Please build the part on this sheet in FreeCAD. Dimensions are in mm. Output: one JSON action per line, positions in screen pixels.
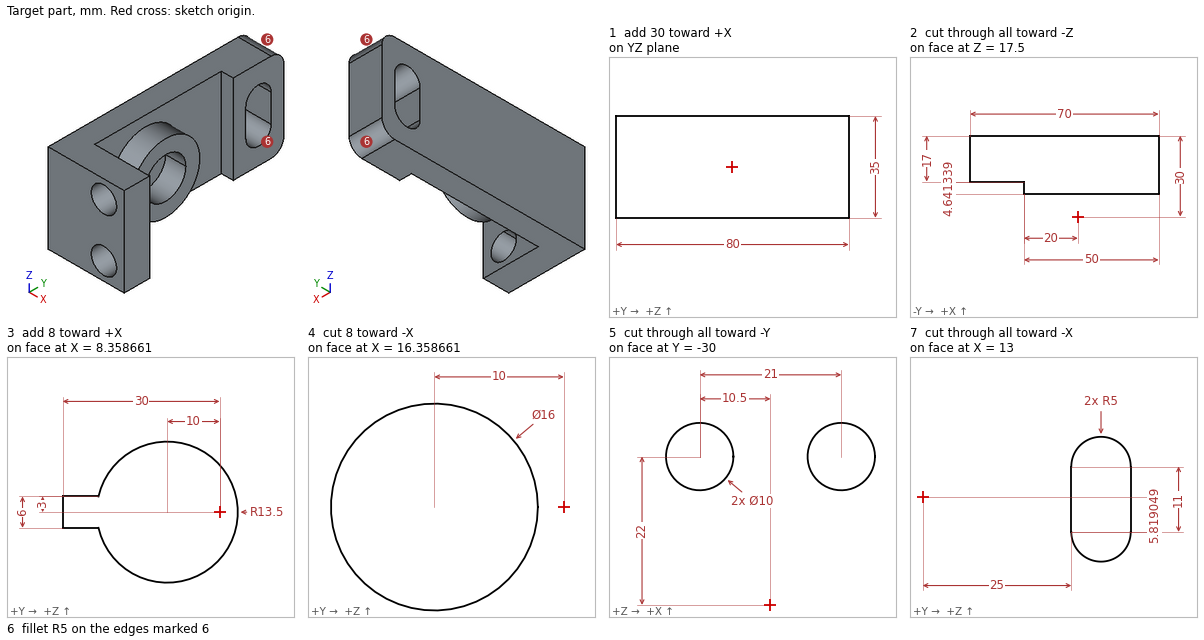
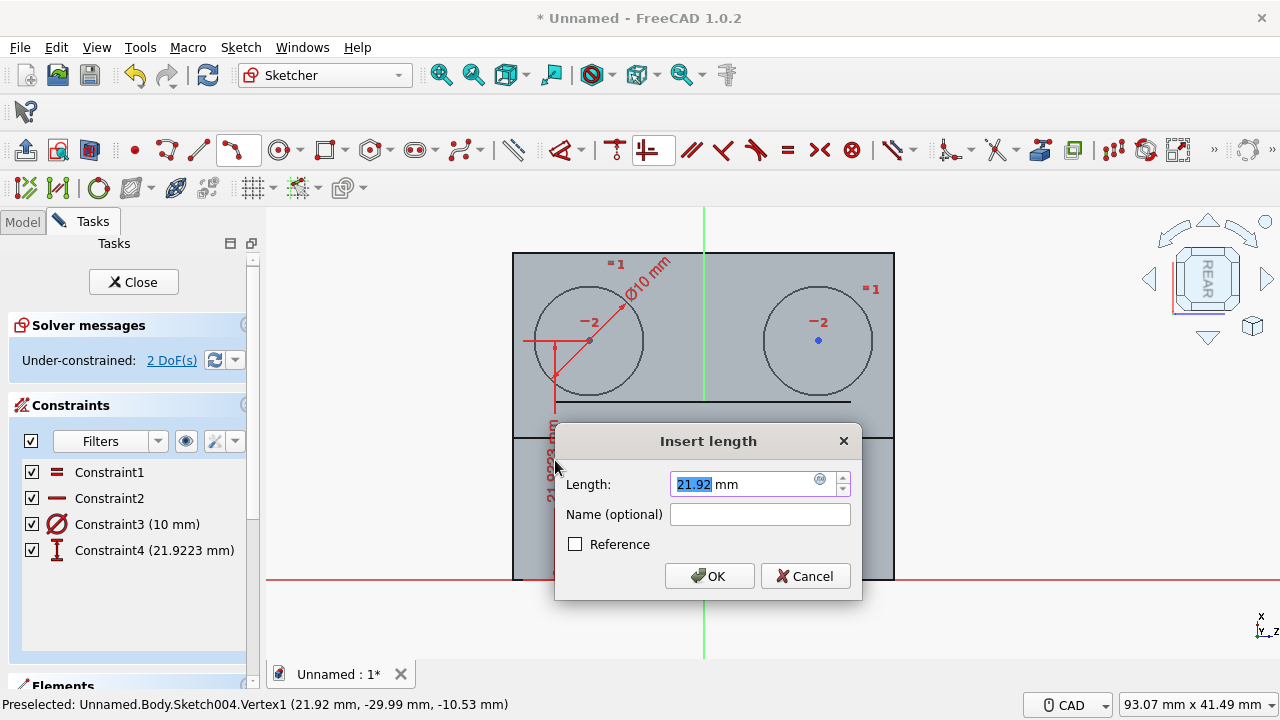
{"action": "type", "text": "22"}
{"action": "key", "text": "Return"}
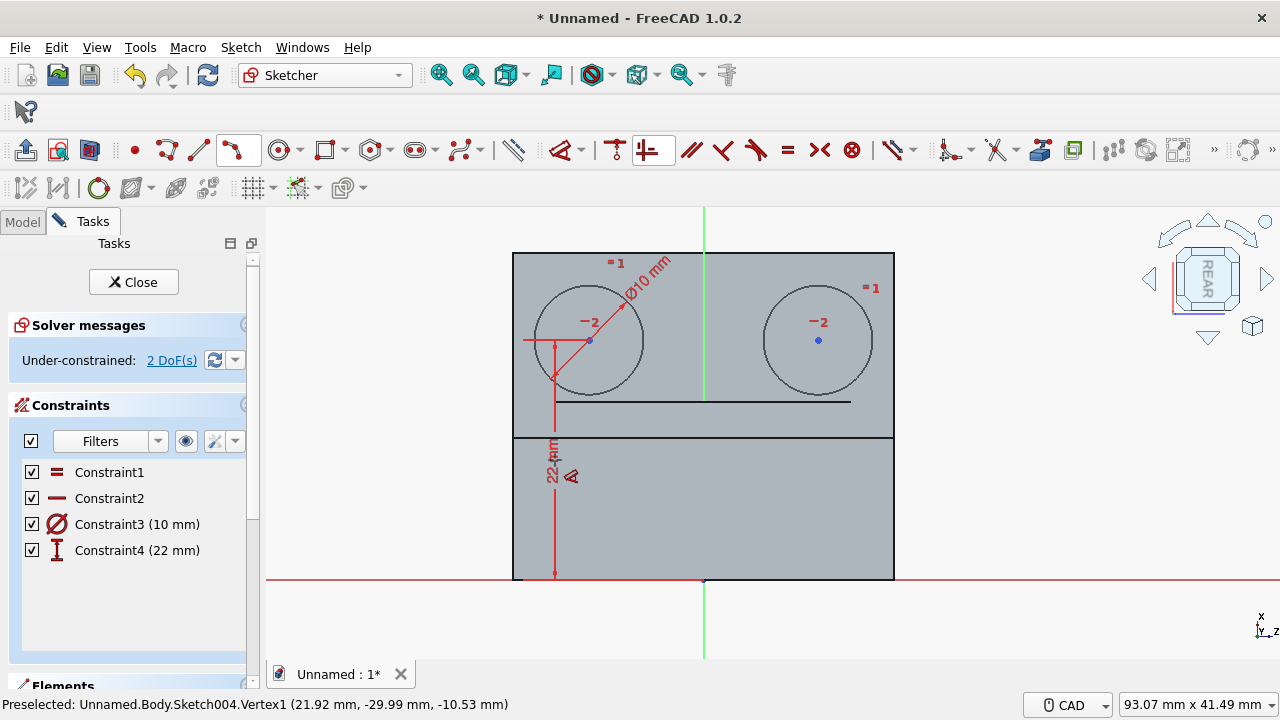
{"action": "left_click", "coordinate": [589, 340]}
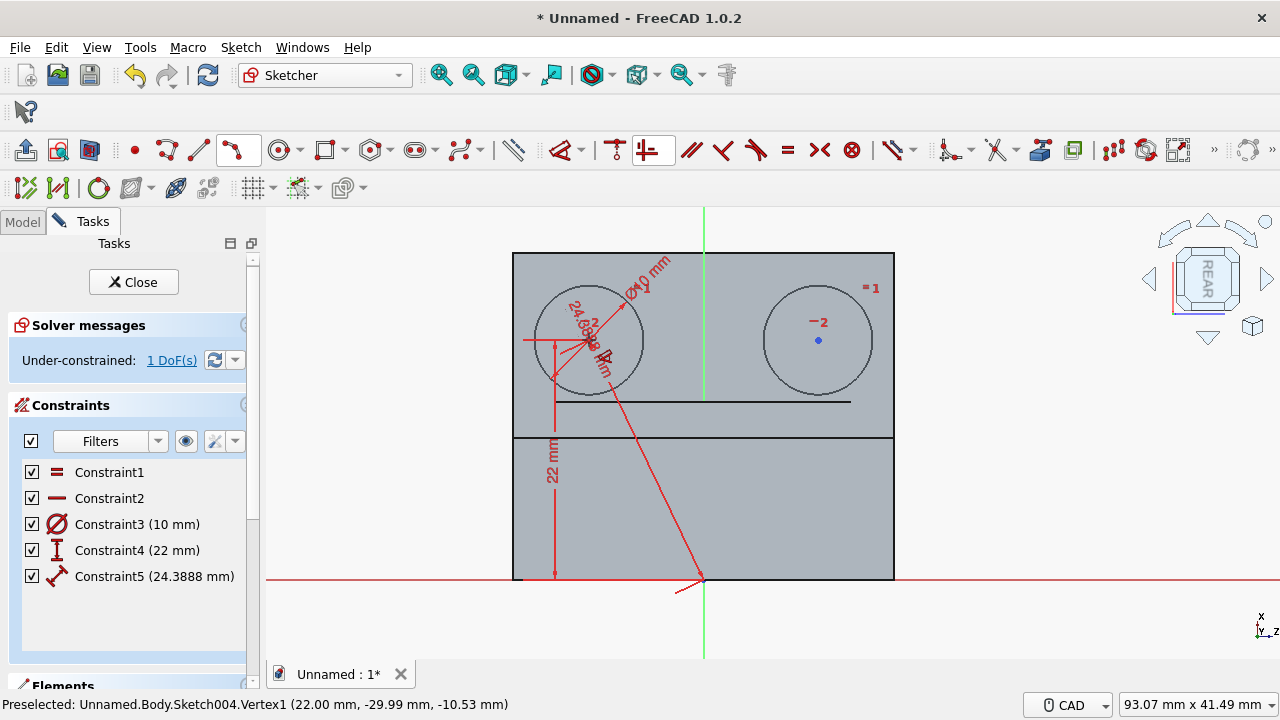
{"action": "left_click", "coordinate": [818, 340]}
{"action": "left_click", "coordinate": [651, 306]}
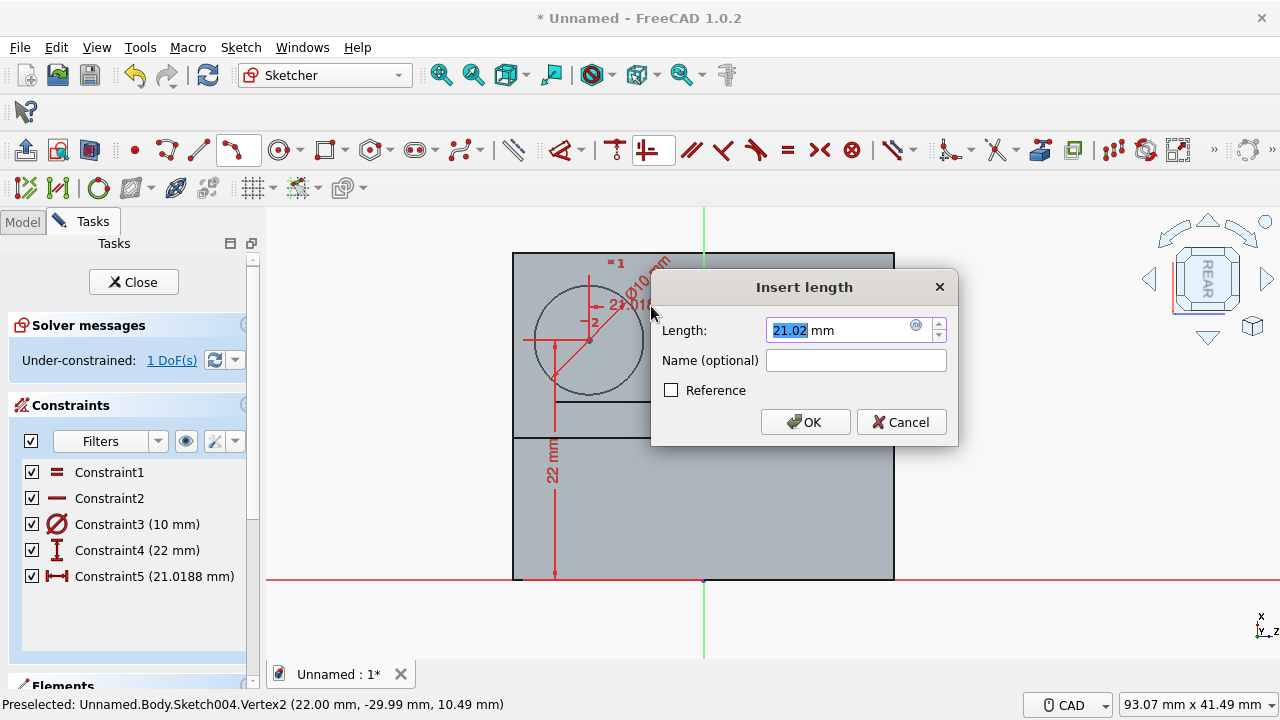
{"action": "type", "text": "21"}
{"action": "key", "text": "Return"}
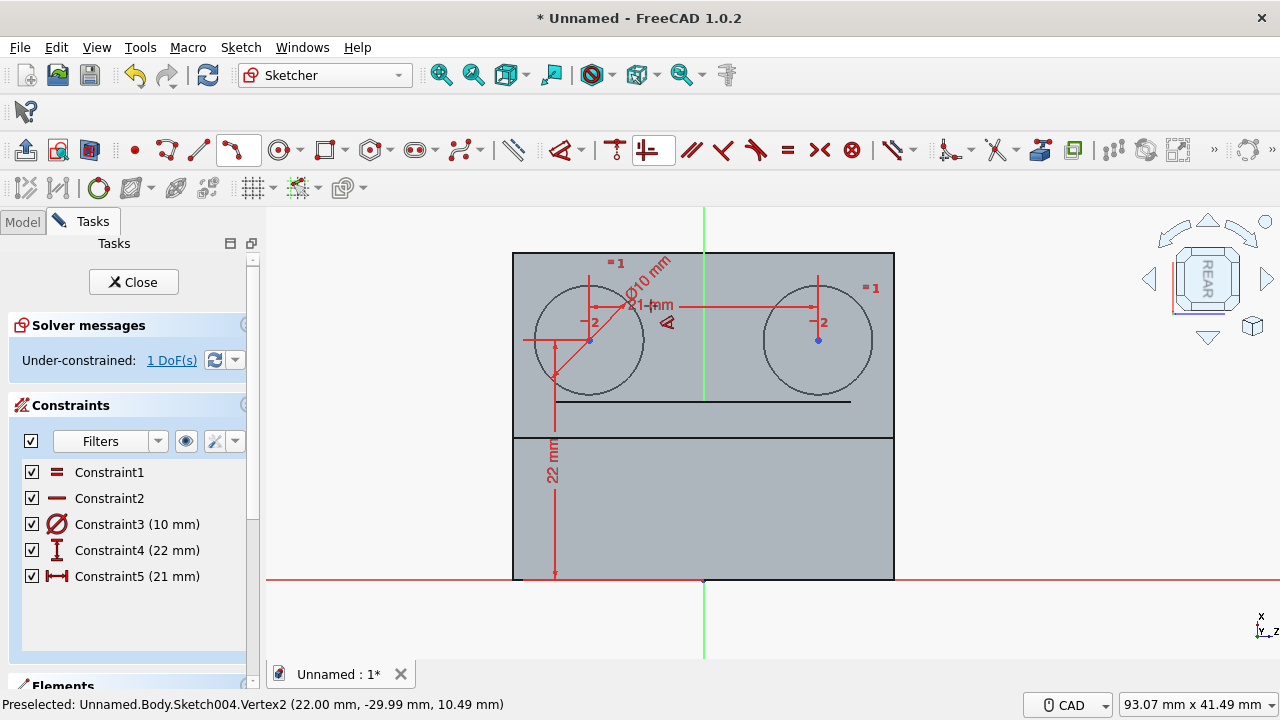
{"action": "left_click", "coordinate": [589, 340]}
{"action": "left_click", "coordinate": [646, 614]}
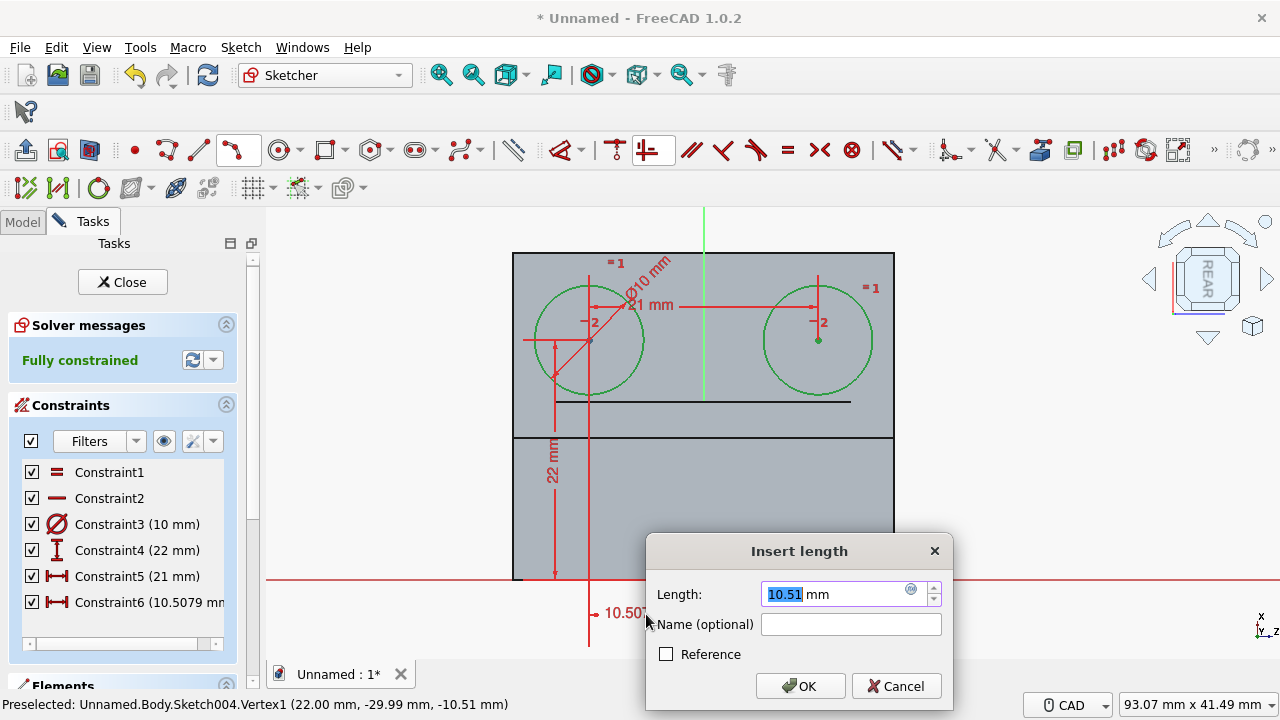
{"action": "type", "text": "10.5"}
{"action": "key", "text": "Return"}
{"action": "key", "text": "Escape"}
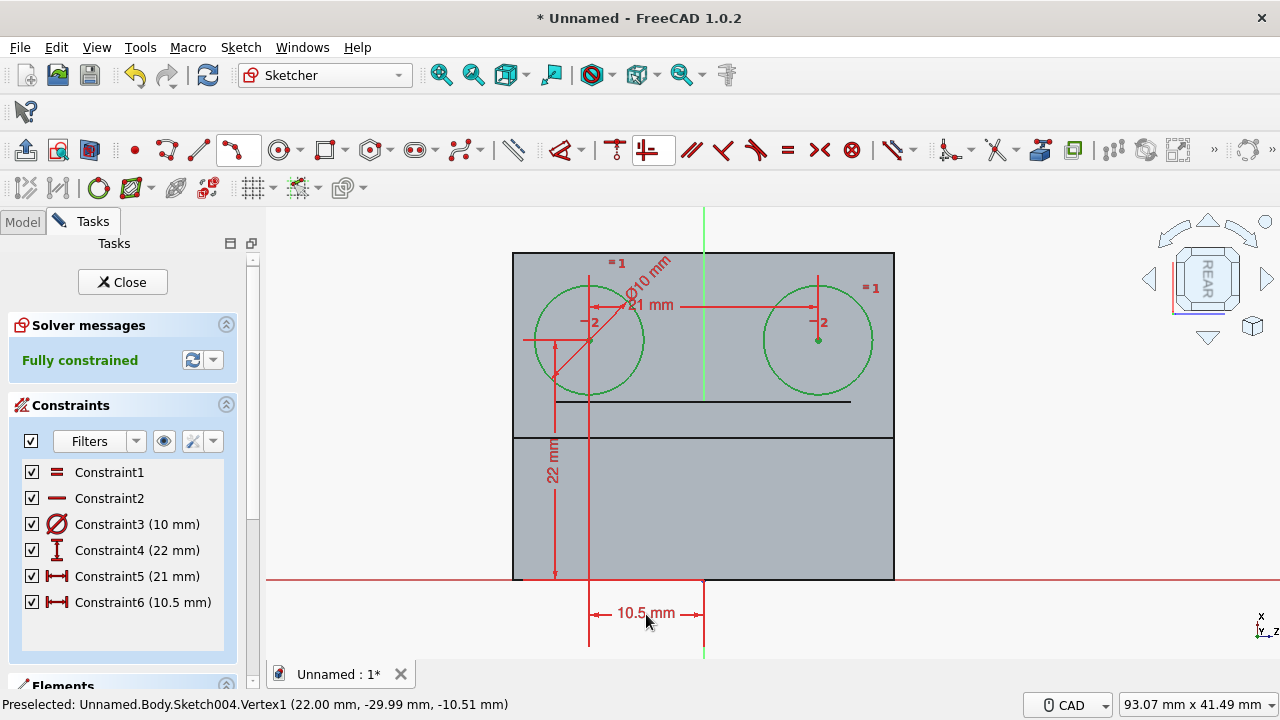
{"action": "left_click", "coordinate": [123, 282]}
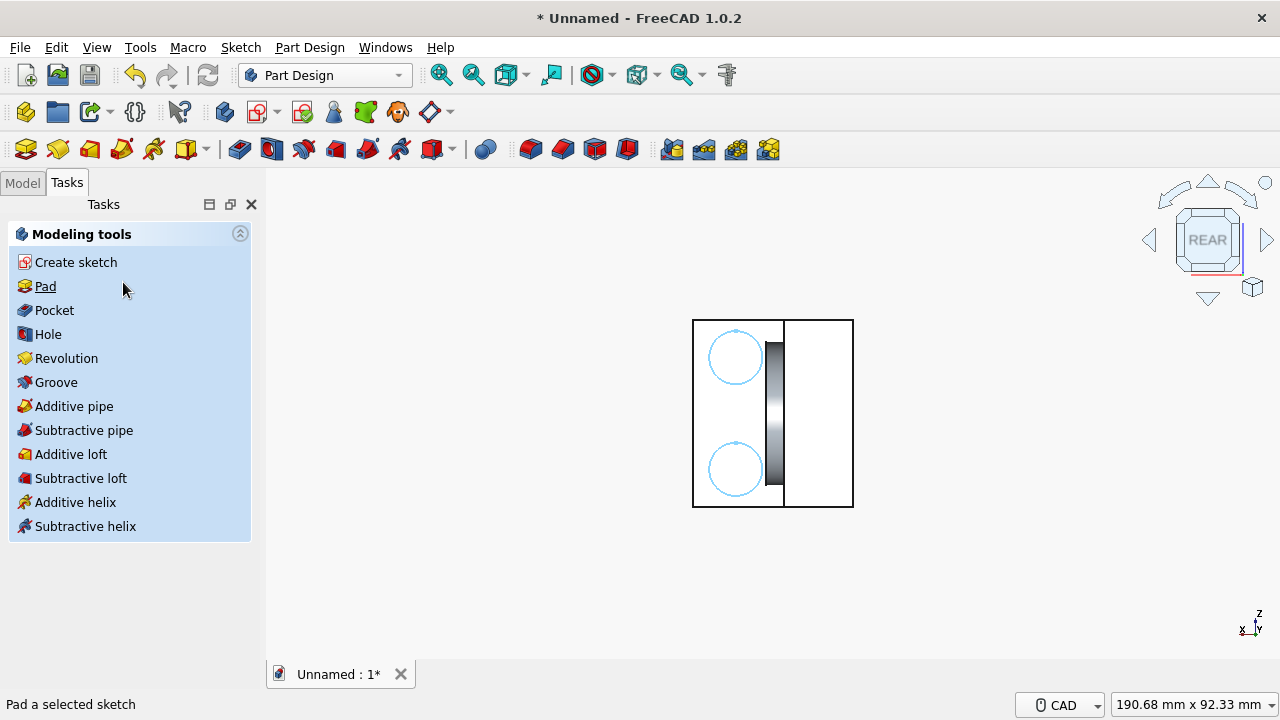
{"action": "left_click", "coordinate": [240, 150]}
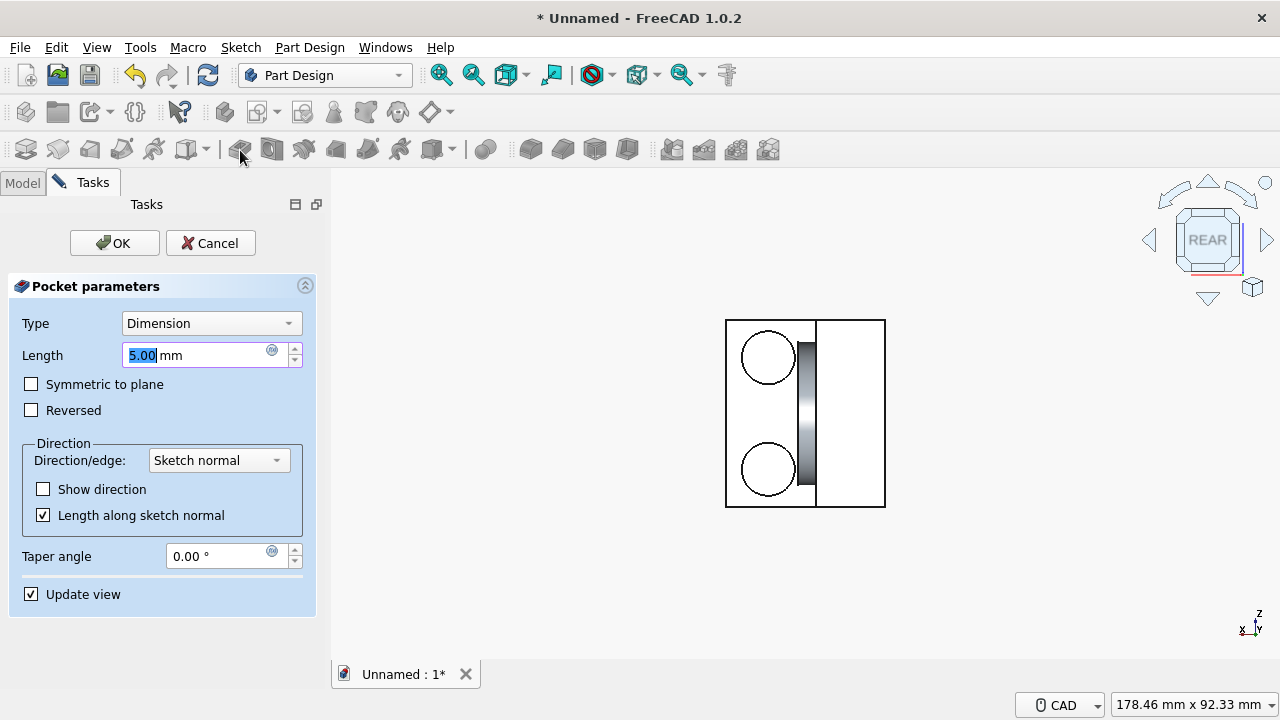
{"action": "left_click", "coordinate": [212, 324]}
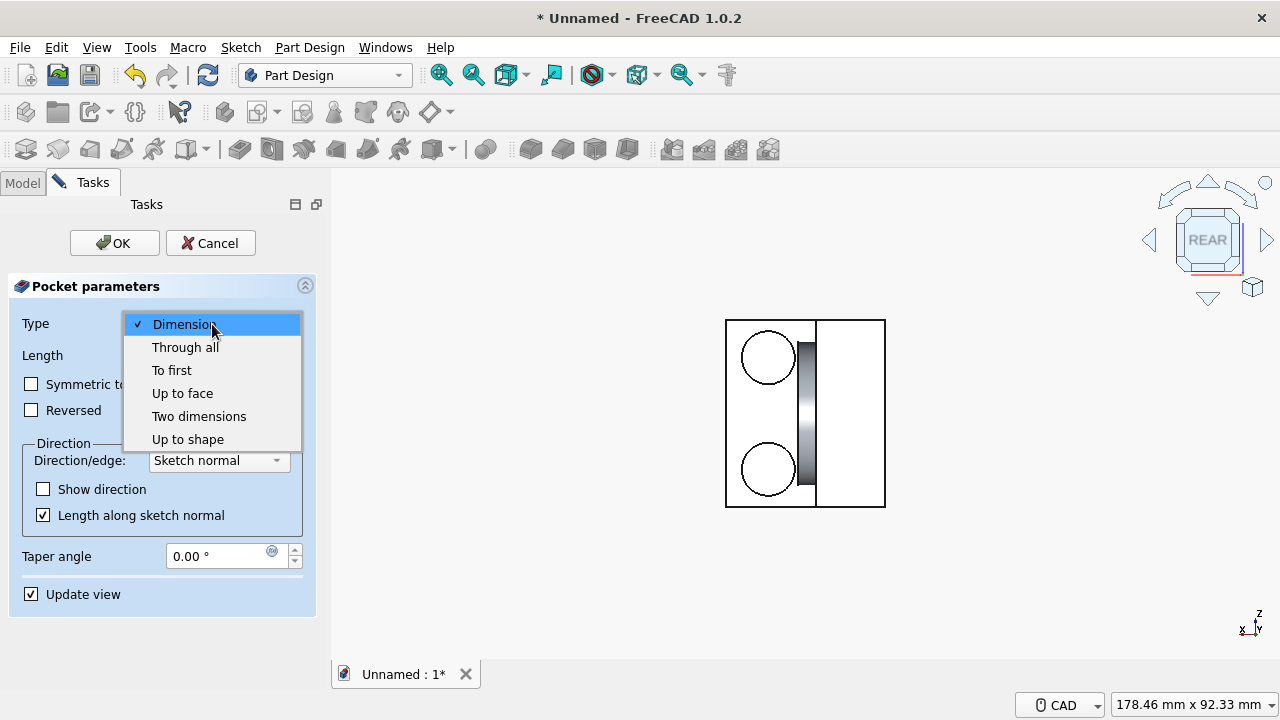
{"action": "left_click", "coordinate": [212, 348]}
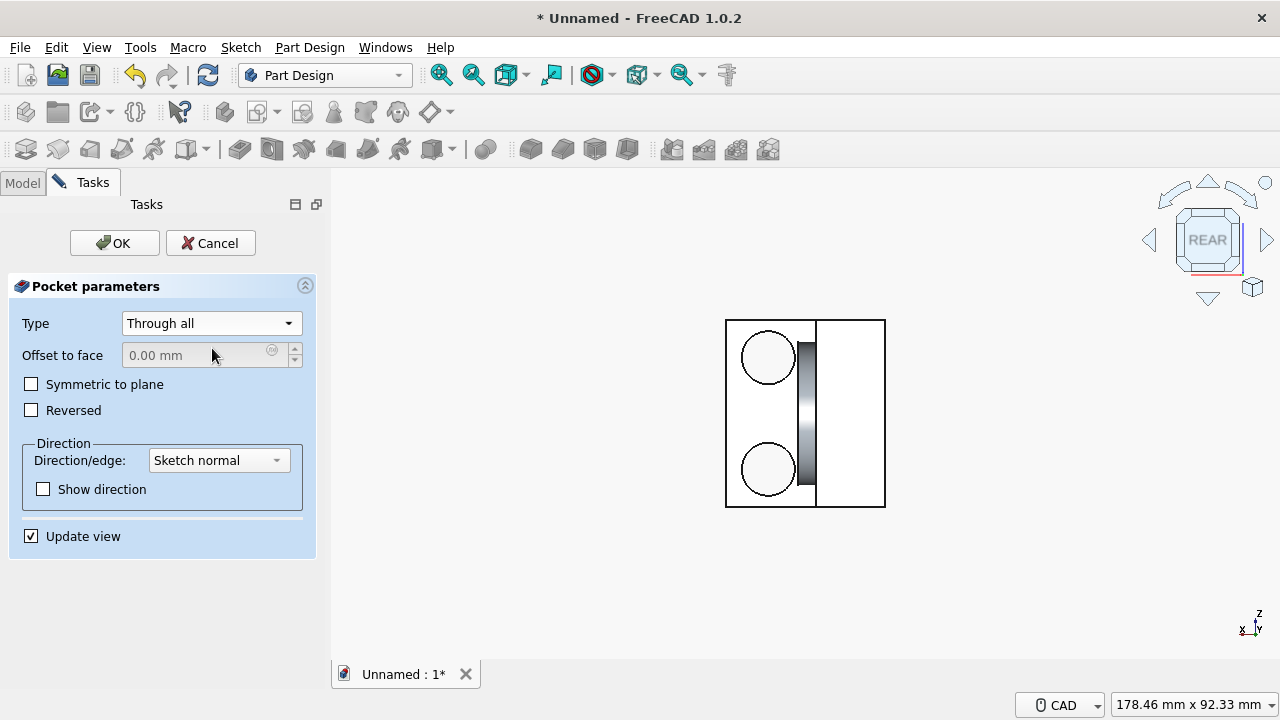
{"action": "left_click", "coordinate": [115, 243]}